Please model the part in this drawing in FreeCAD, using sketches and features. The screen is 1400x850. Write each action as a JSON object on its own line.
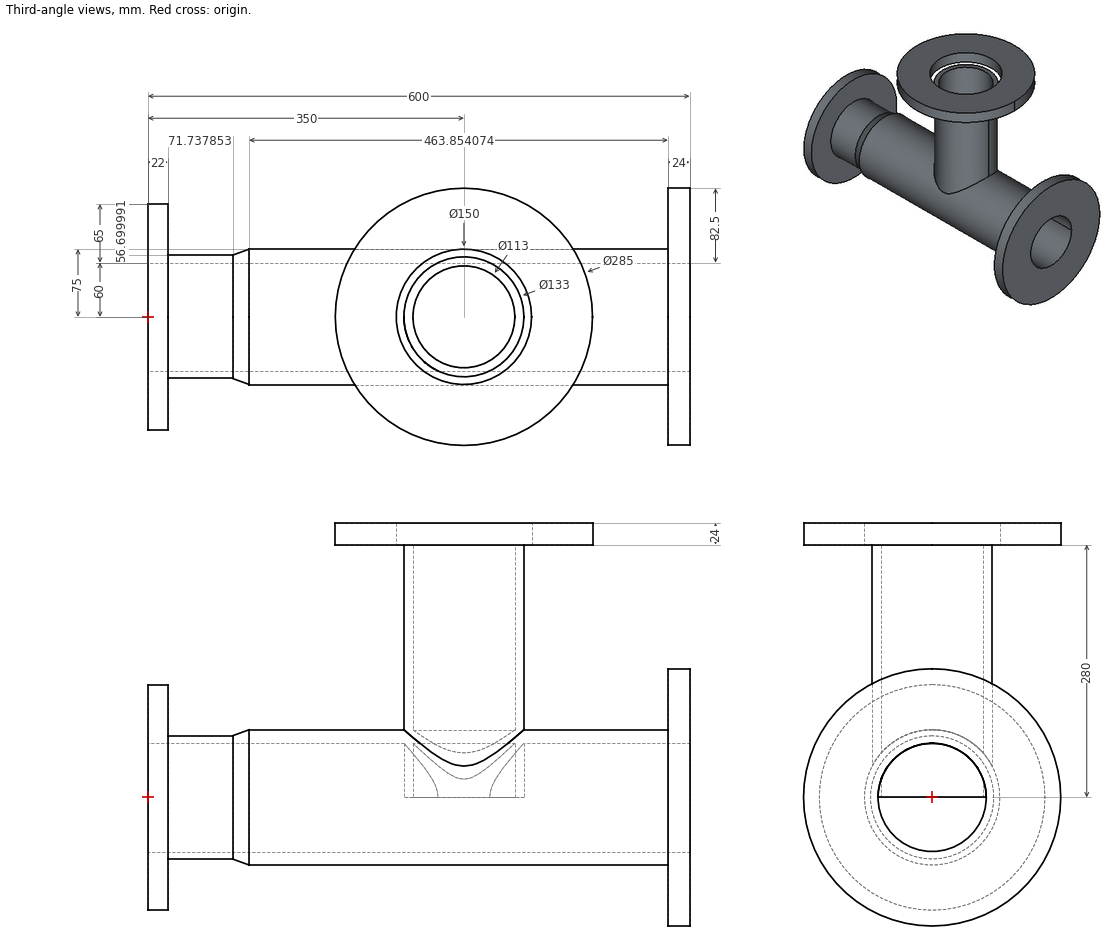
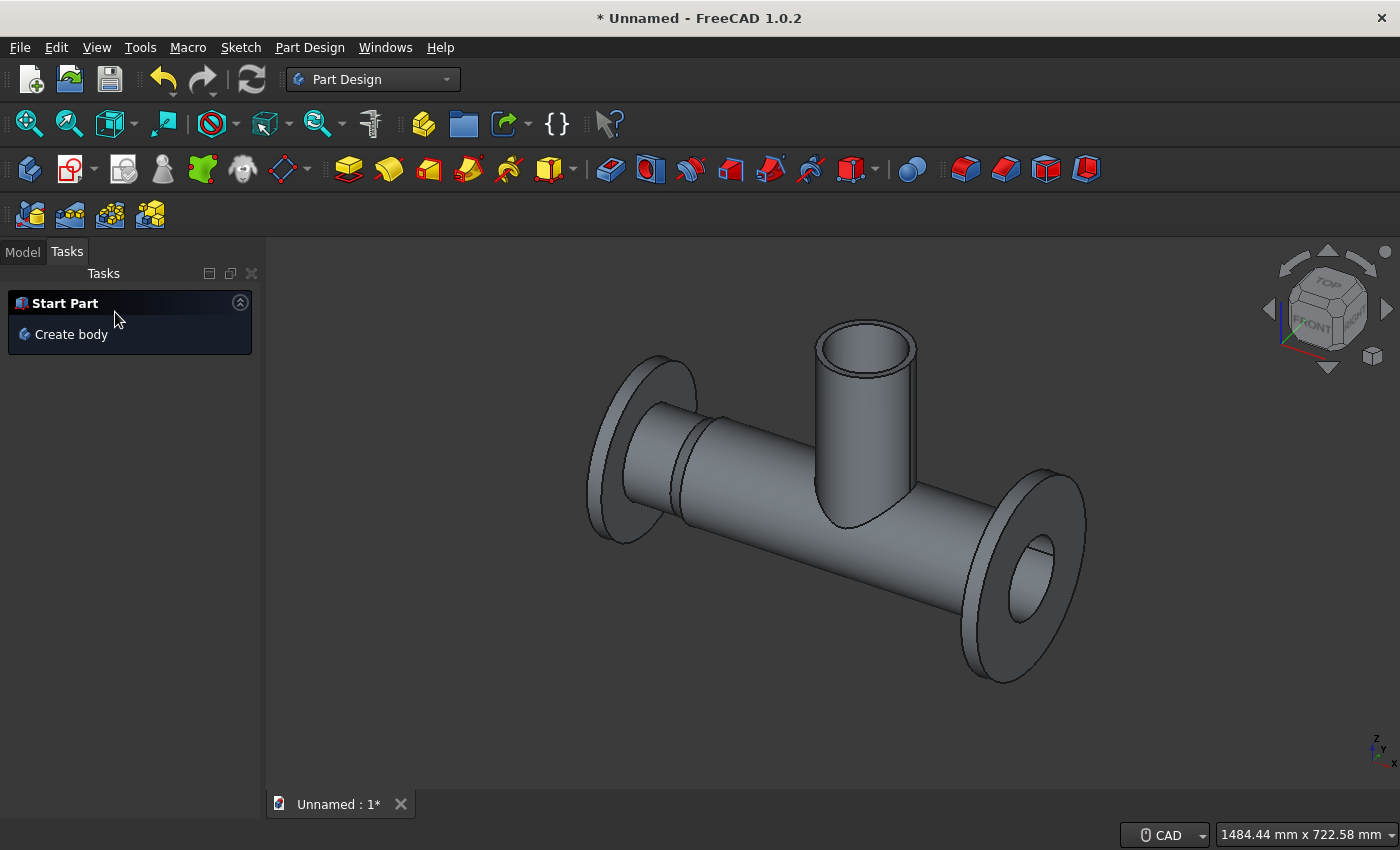
{"action": "left_click", "coordinate": [30, 124]}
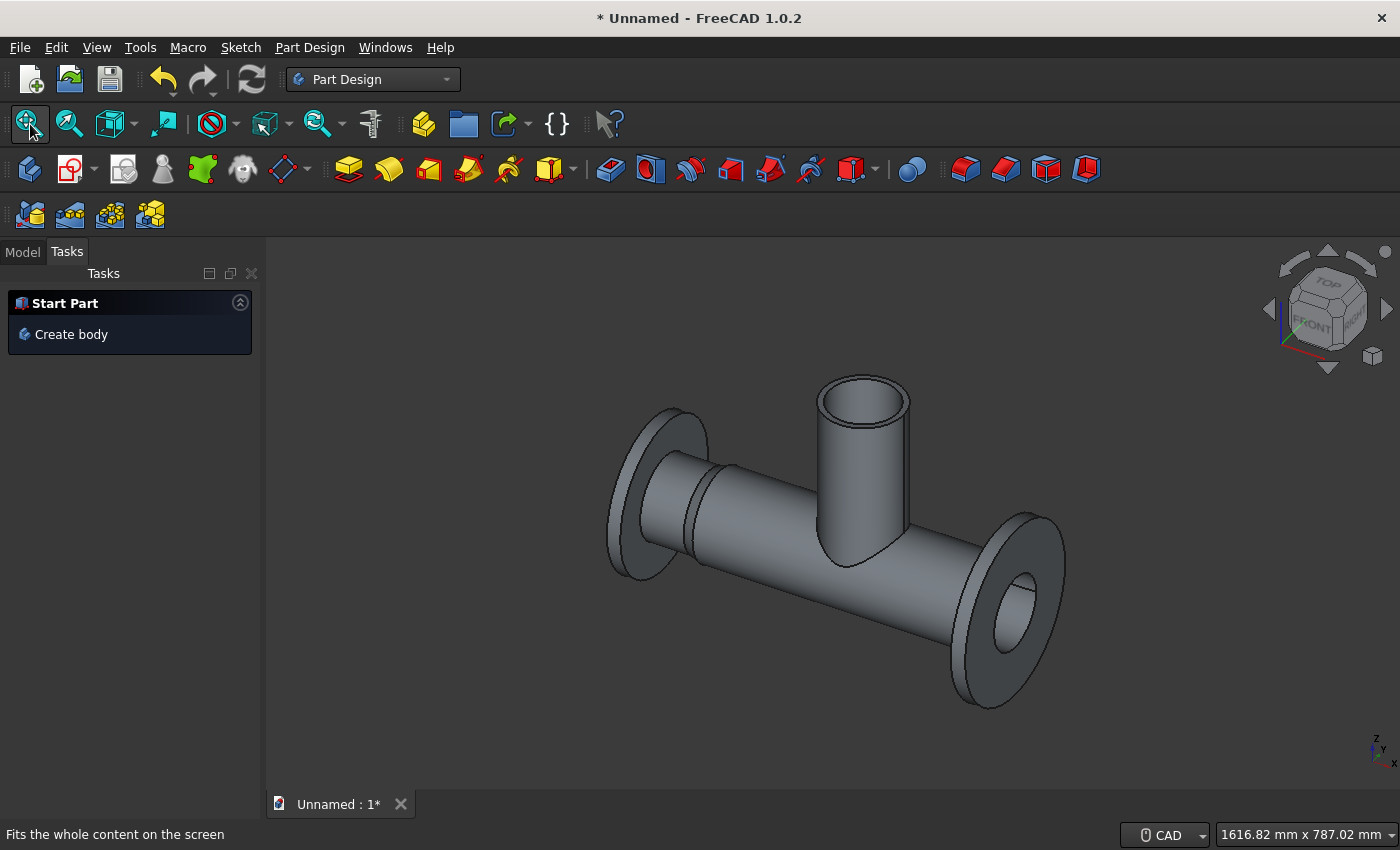
{"action": "left_click", "coordinate": [30, 170]}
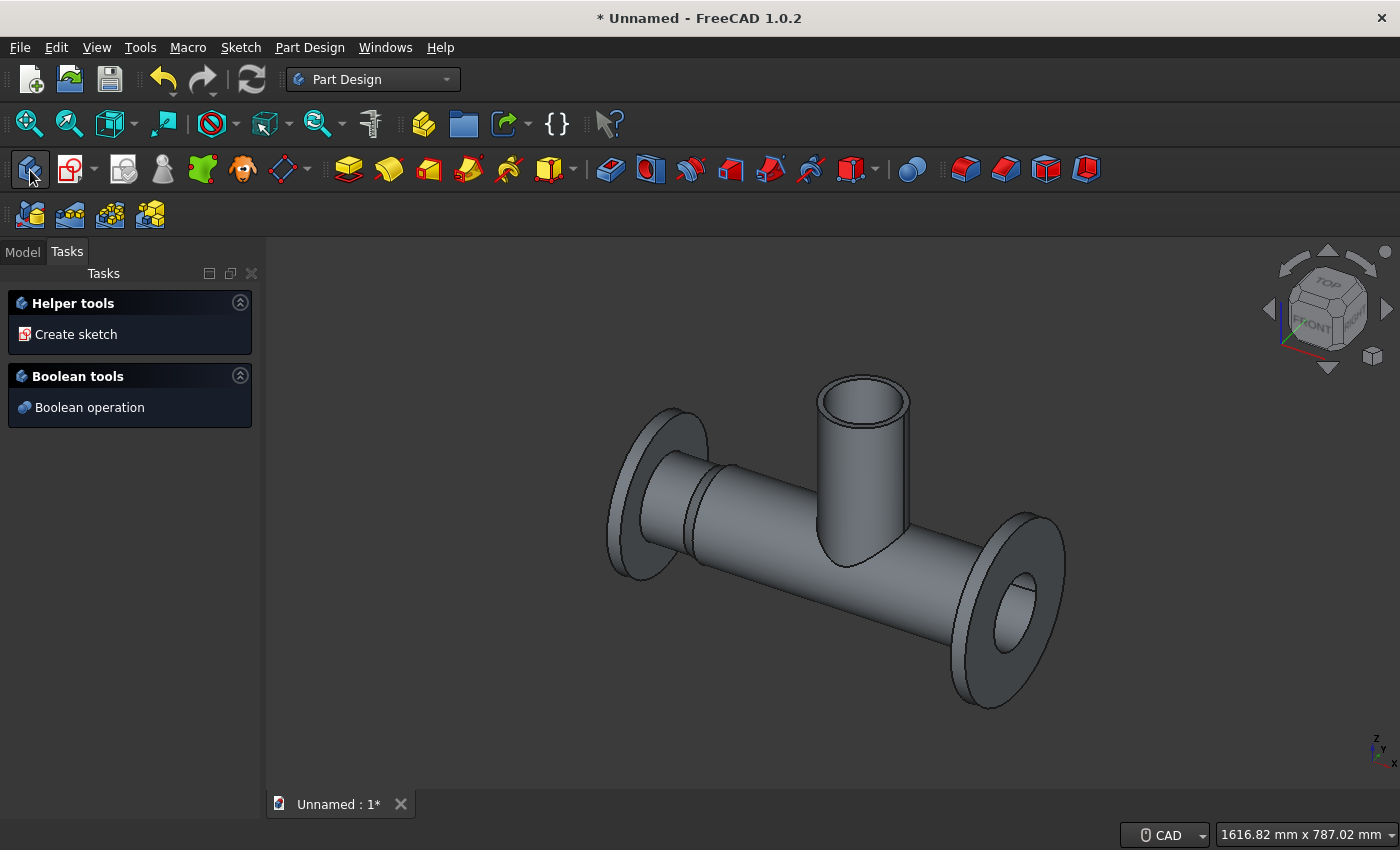
{"action": "left_click", "coordinate": [23, 251]}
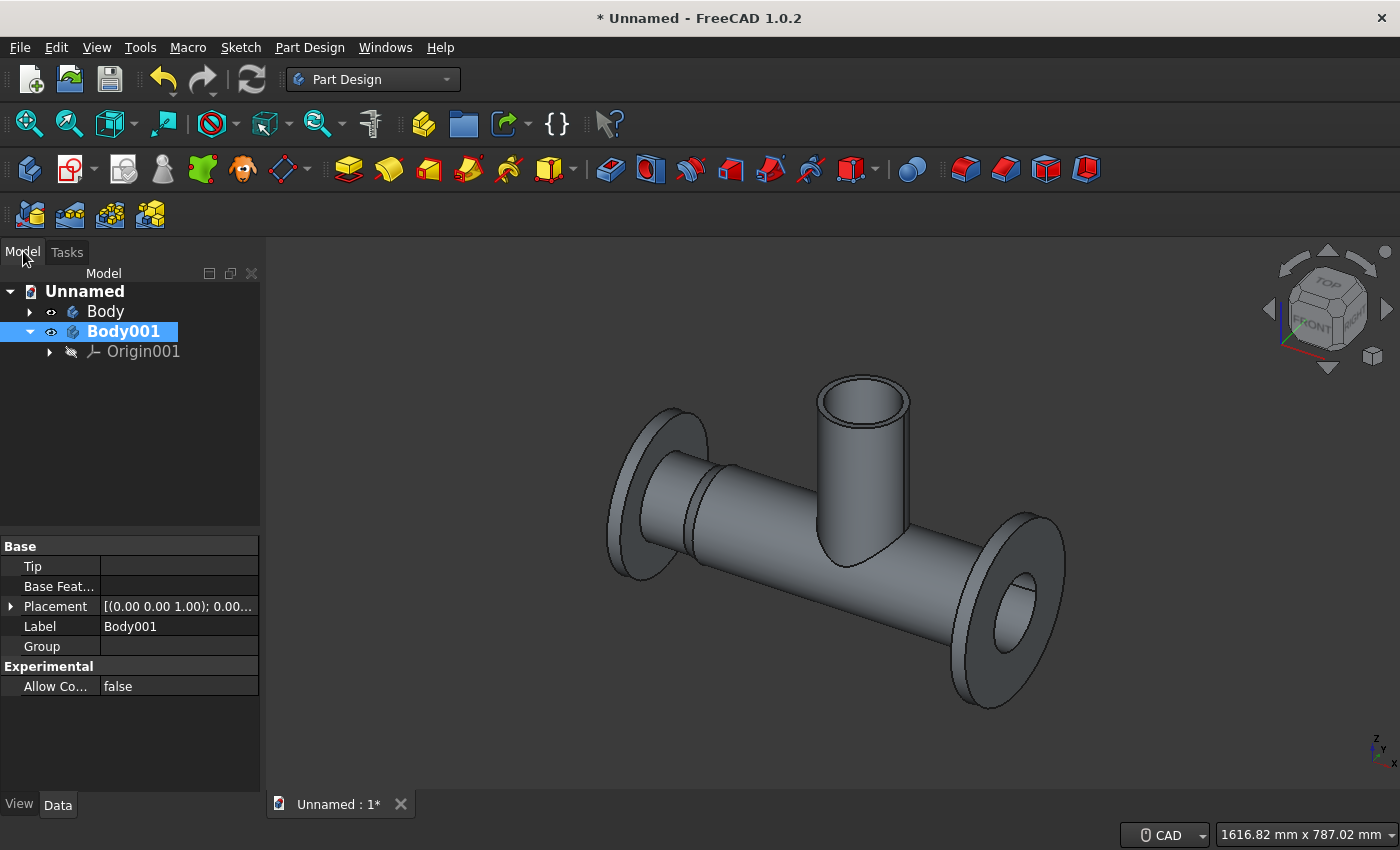
{"action": "left_click", "coordinate": [50, 352]}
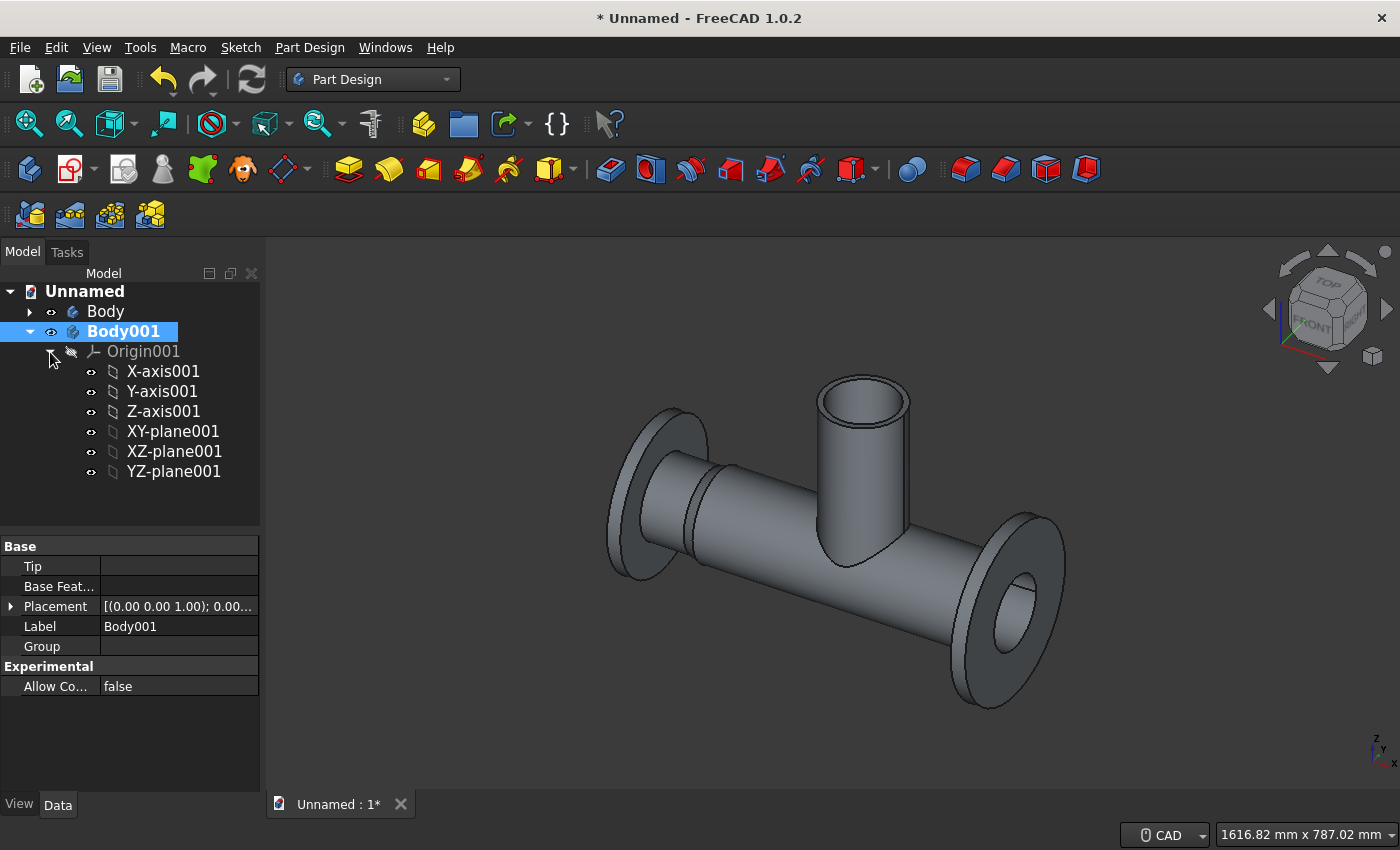
{"action": "left_click", "coordinate": [136, 432]}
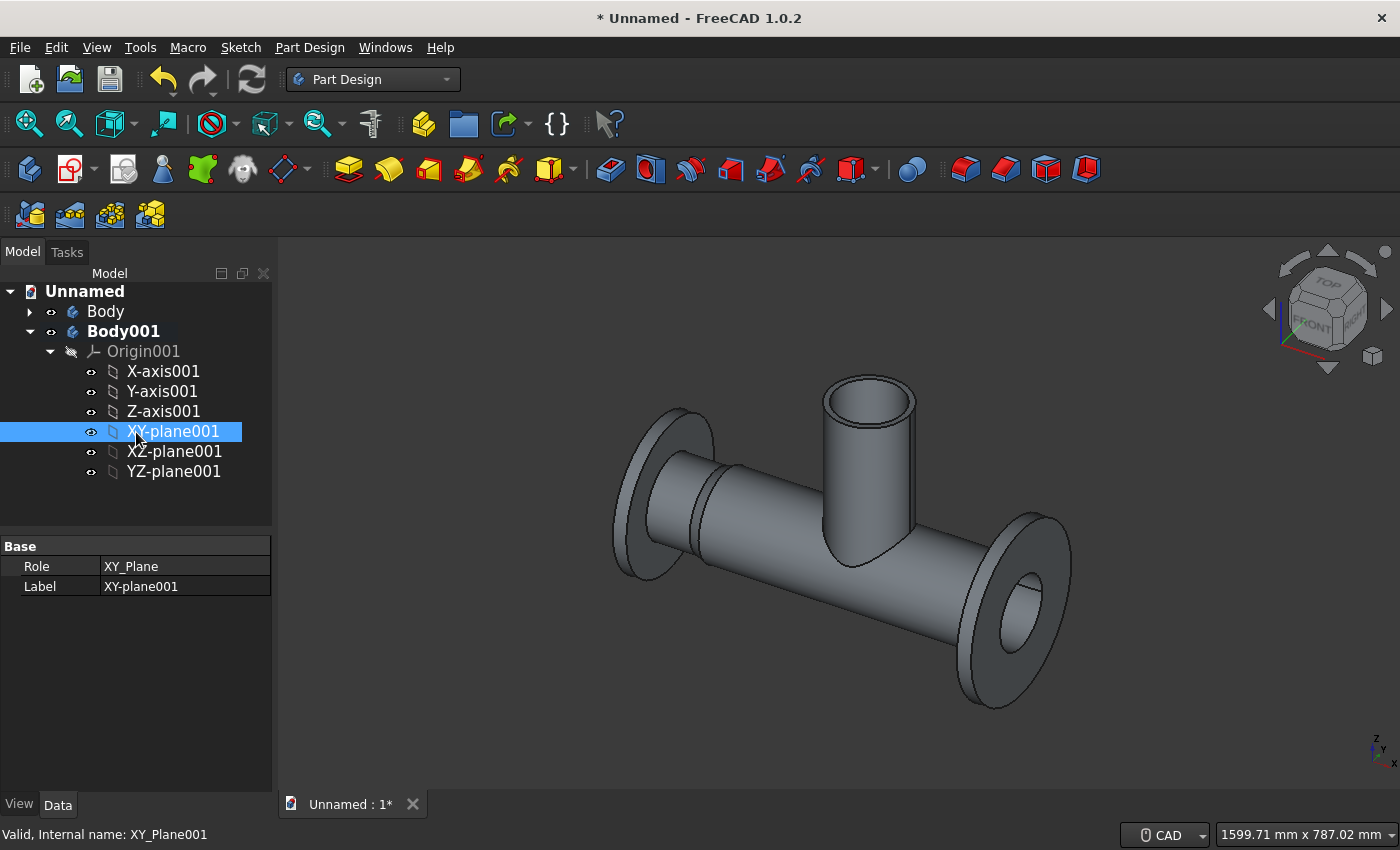
{"action": "left_click", "coordinate": [284, 170]}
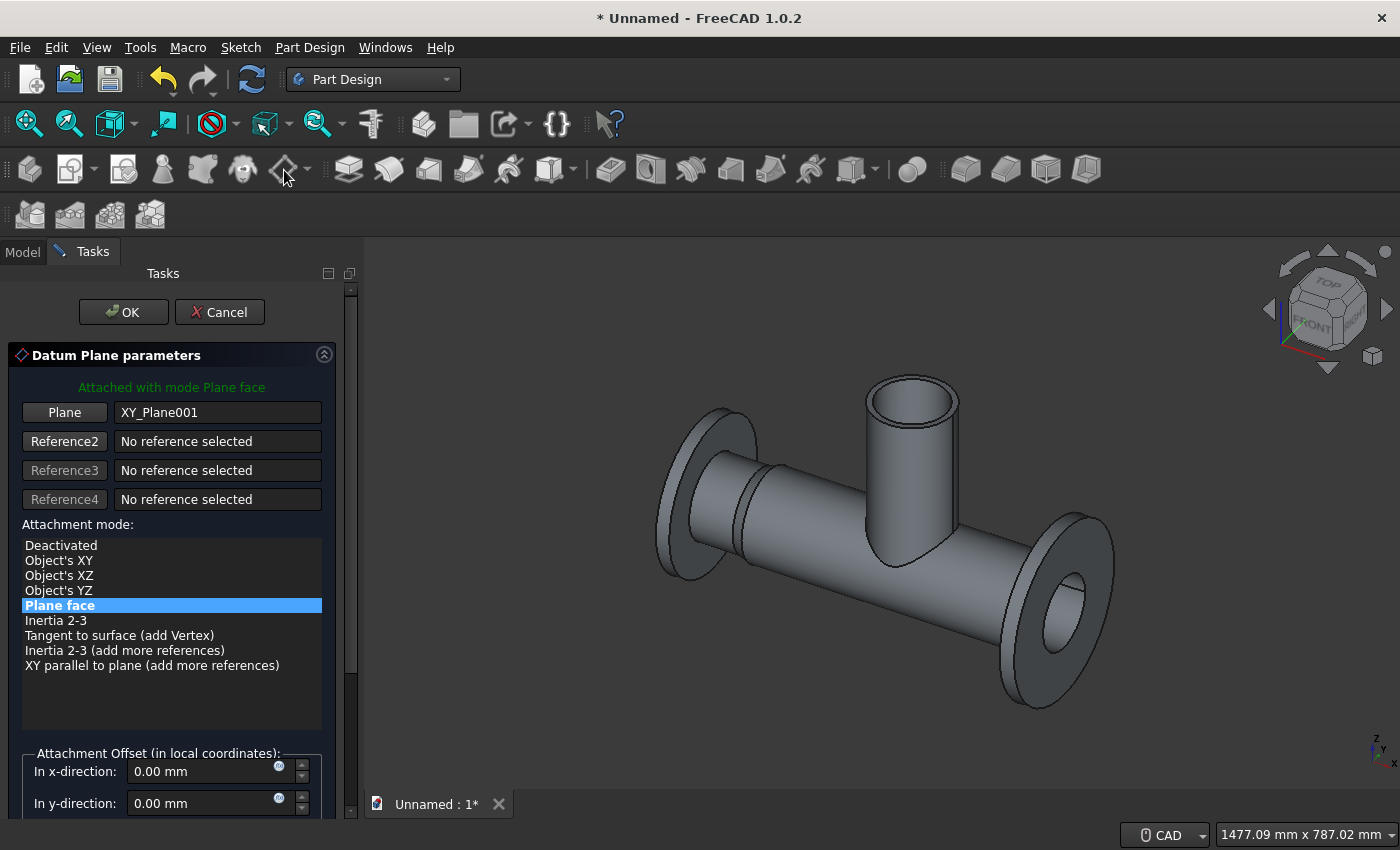
{"action": "scroll", "coordinate": [351, 550], "scroll_direction": "down", "scroll_amount": 2}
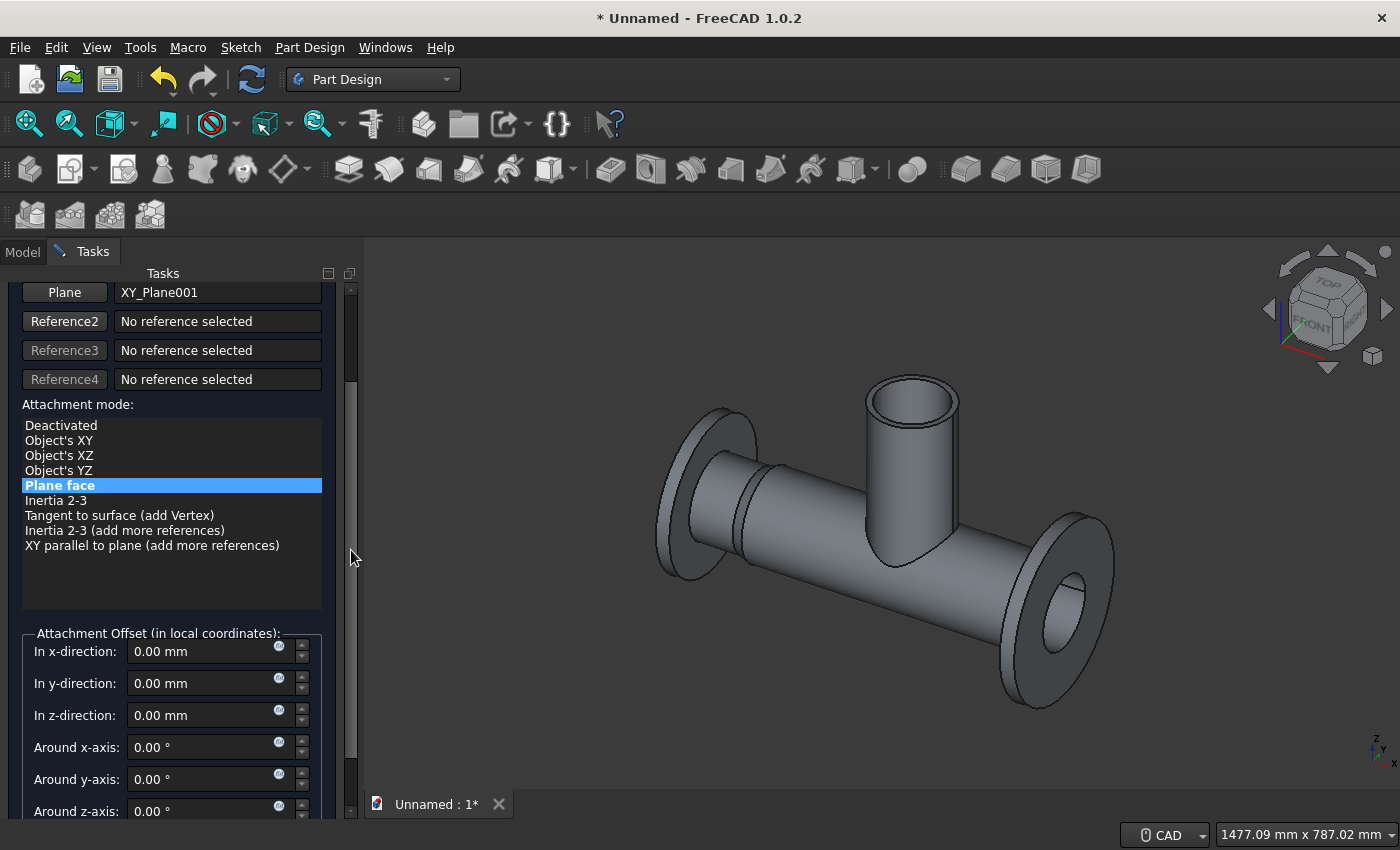
{"action": "triple_click", "coordinate": [210, 715]}